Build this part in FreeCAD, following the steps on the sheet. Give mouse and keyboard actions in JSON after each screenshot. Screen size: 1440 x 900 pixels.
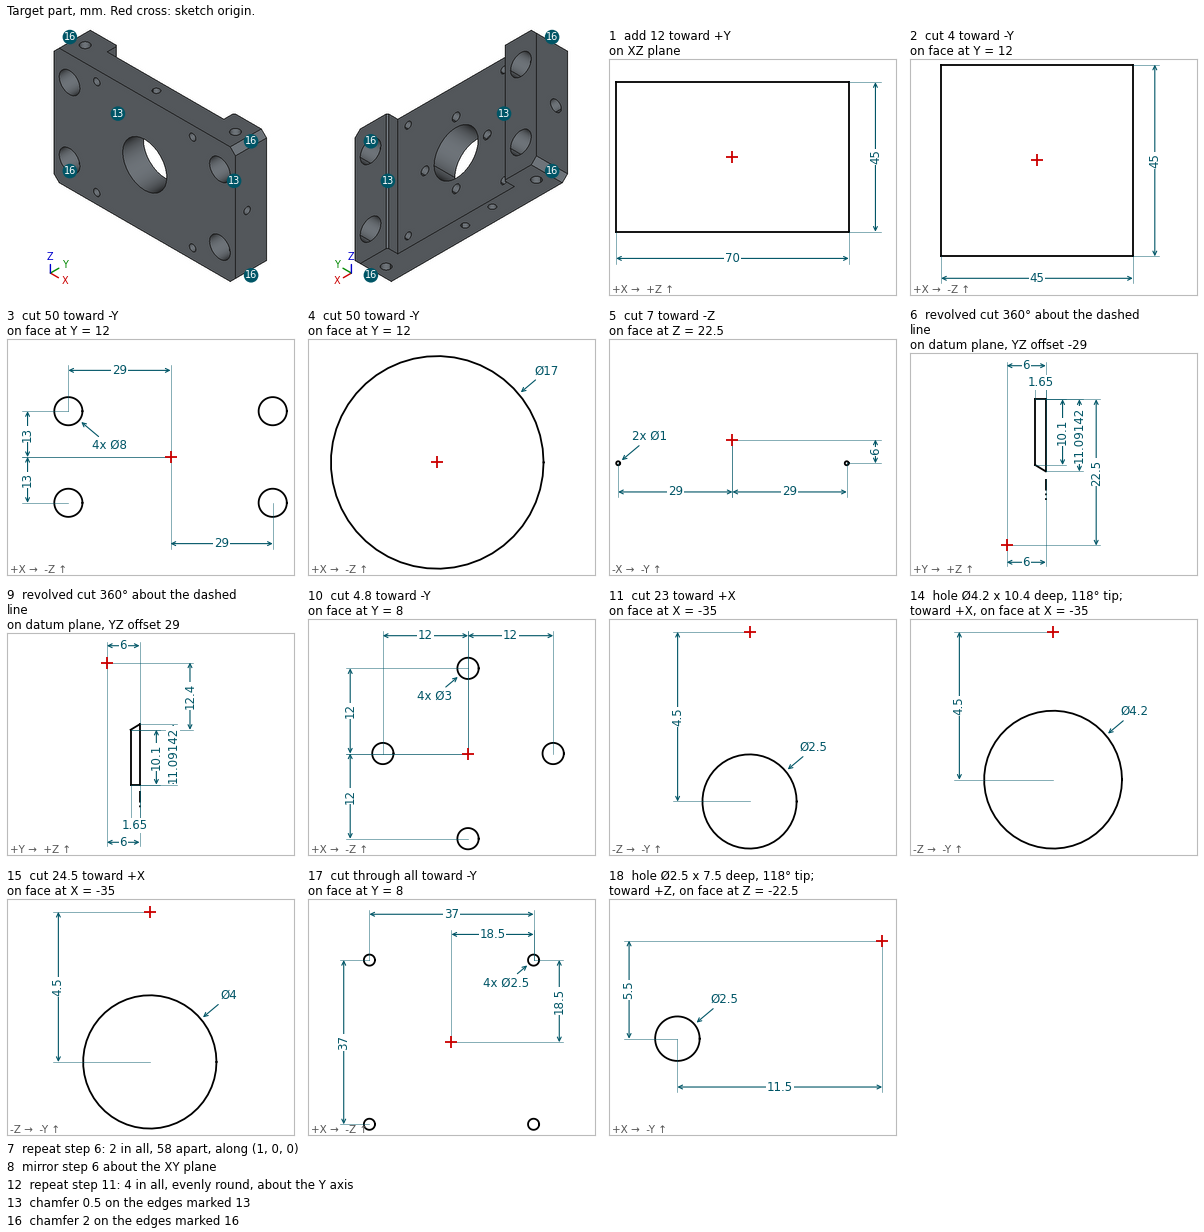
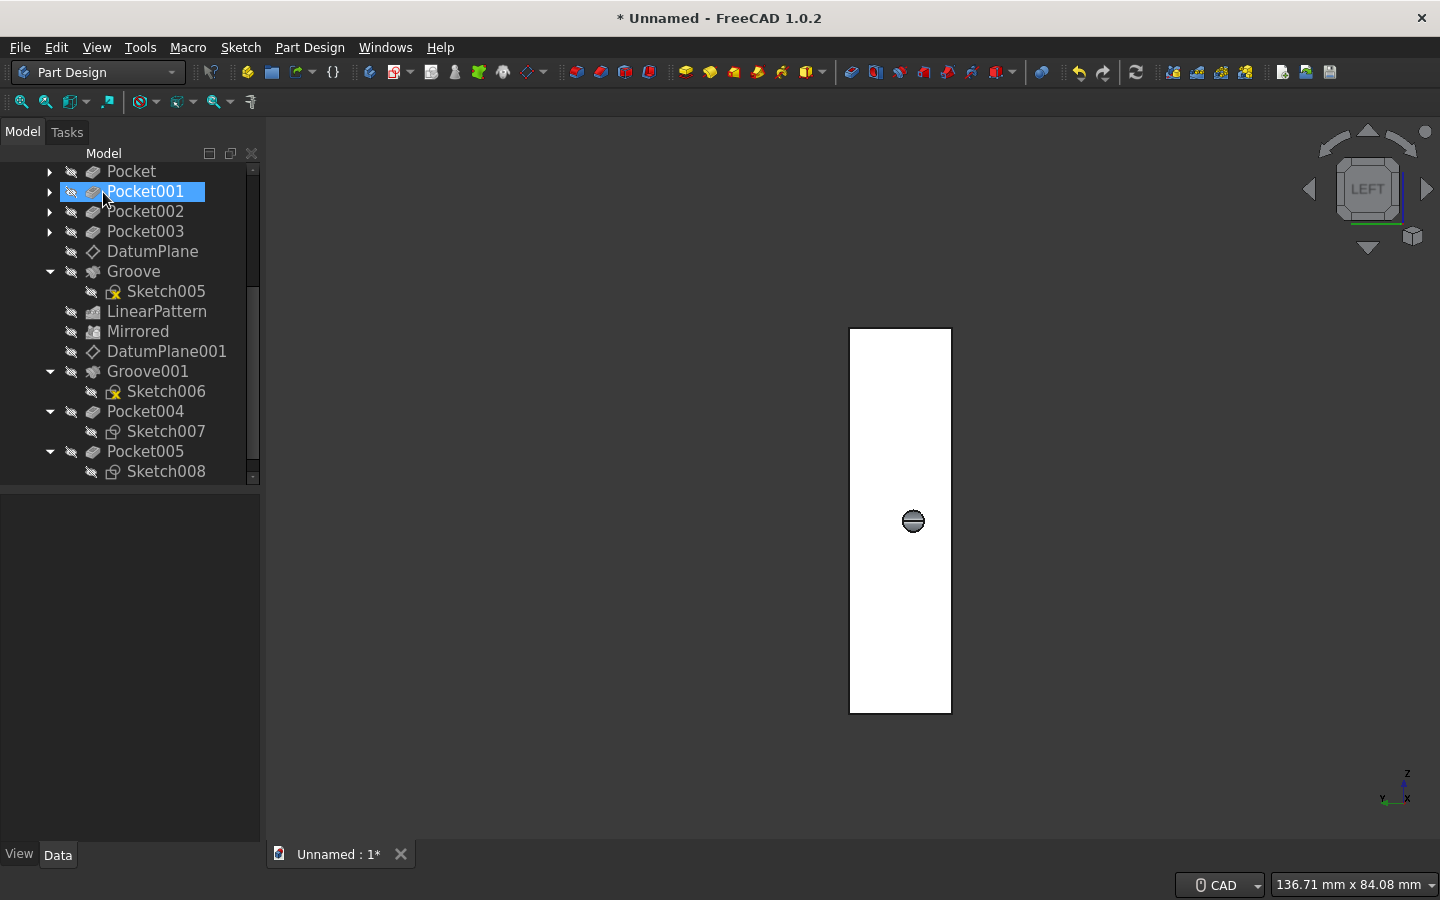
{"action": "key", "text": "0"}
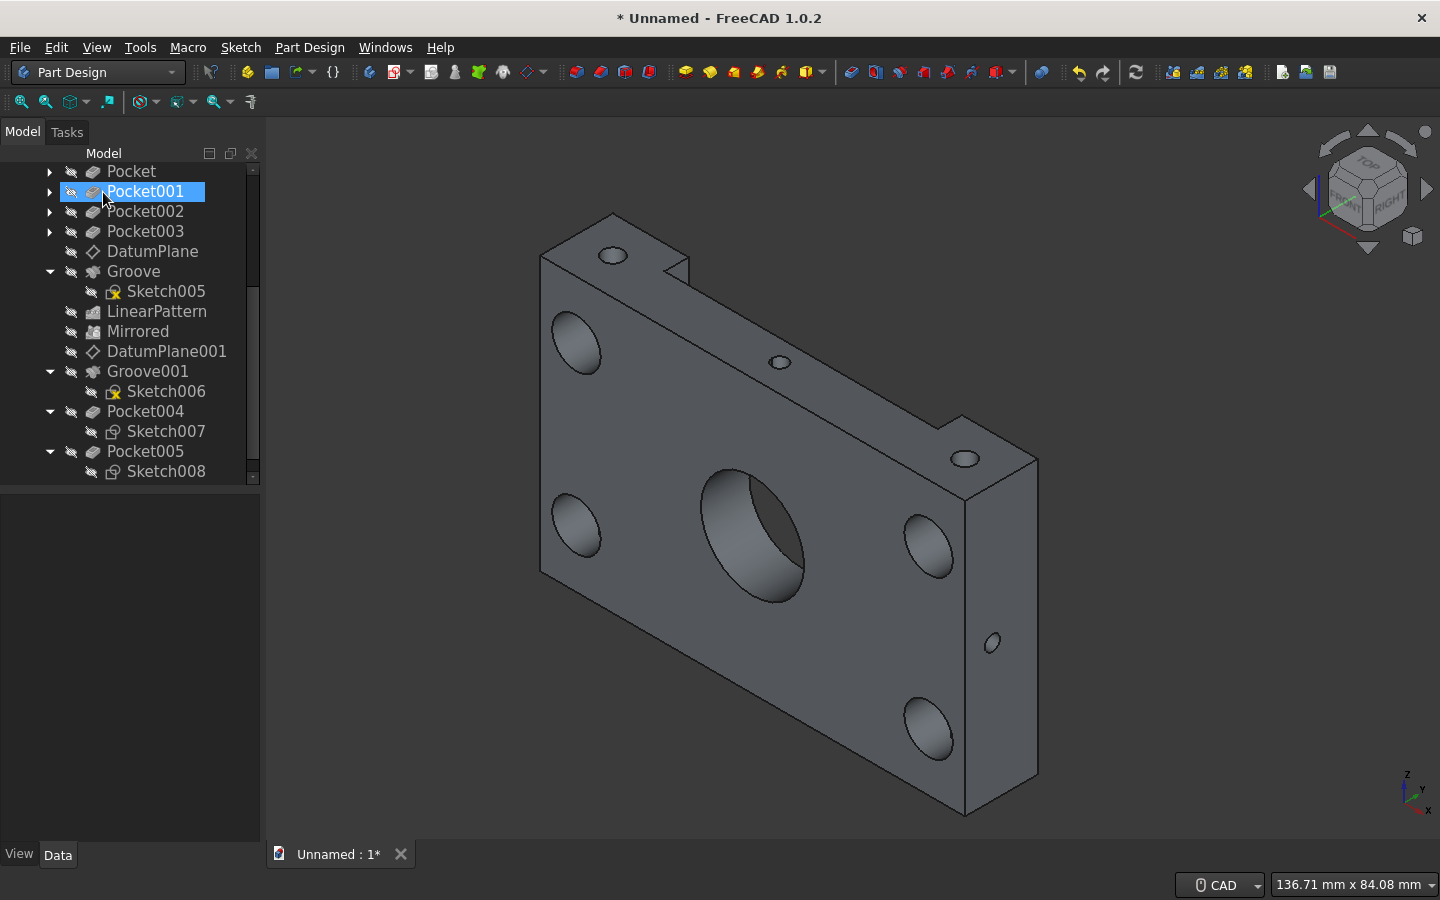
{"action": "key", "text": "2"}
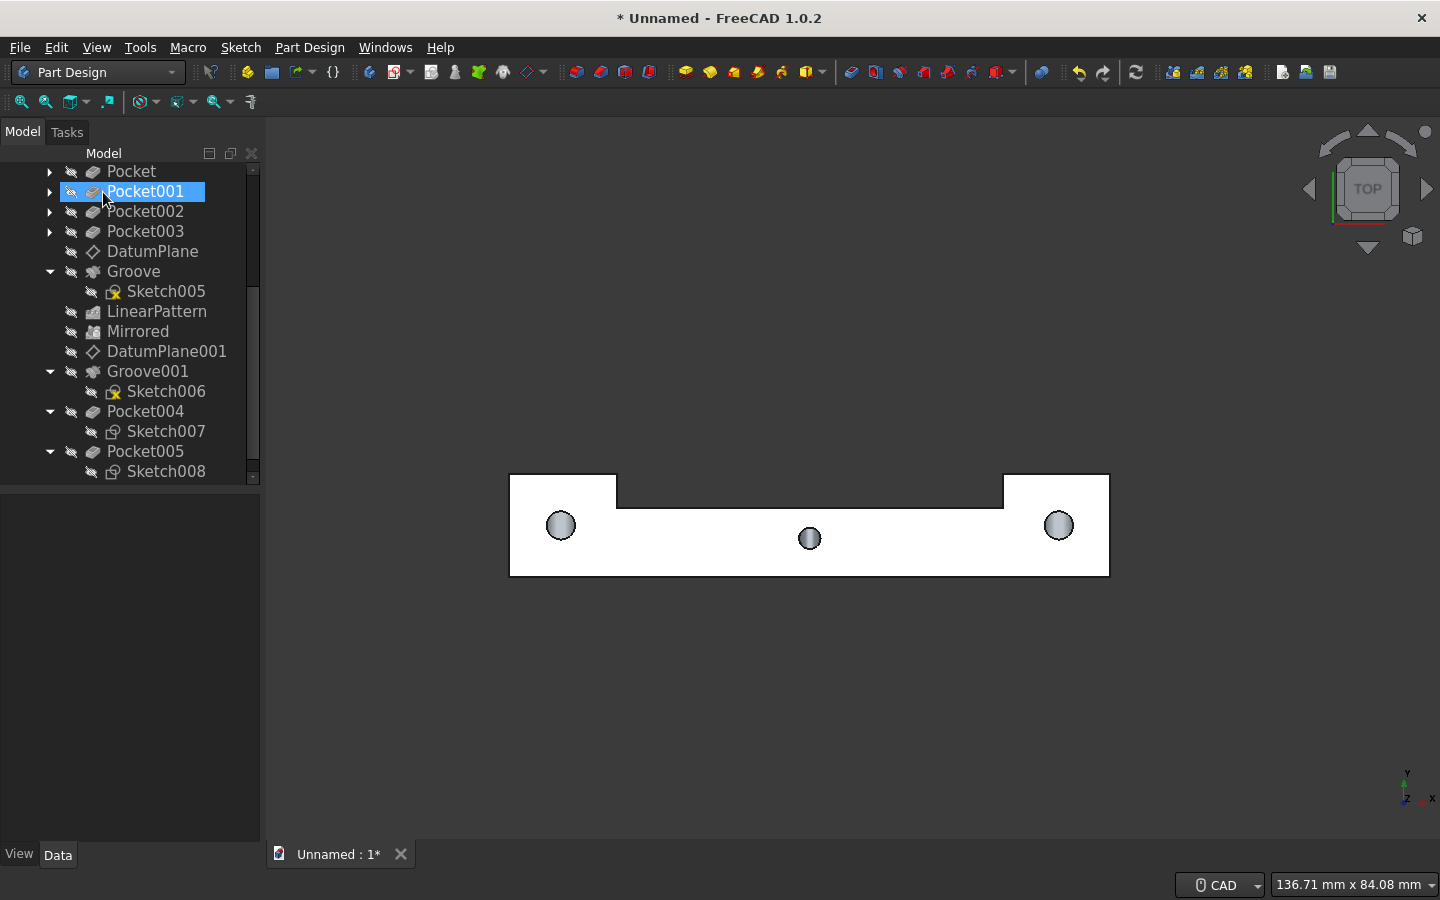
{"action": "key", "text": "1"}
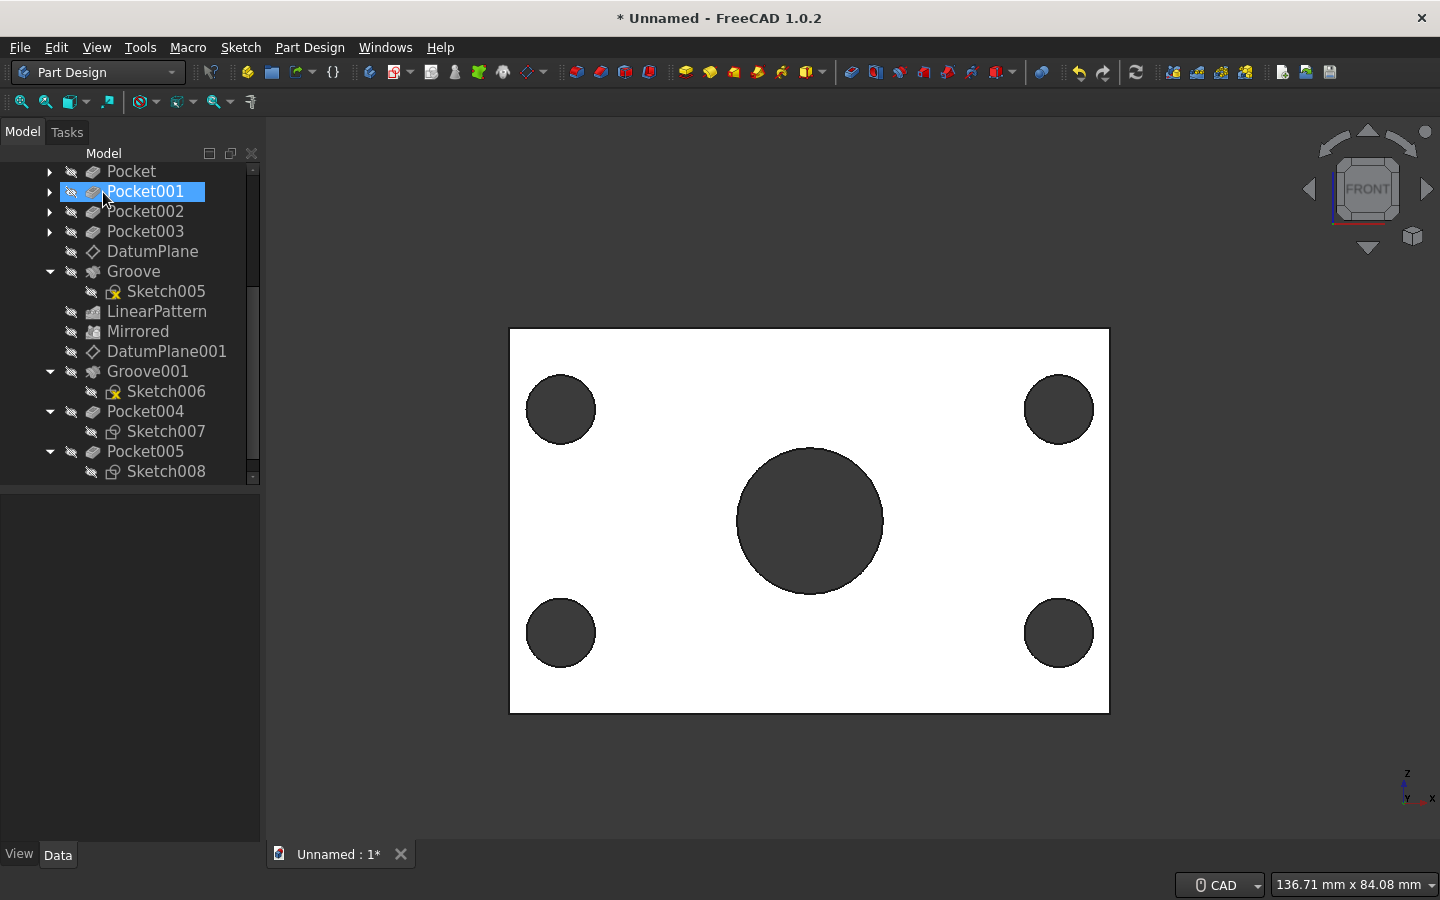
{"action": "key", "text": "3"}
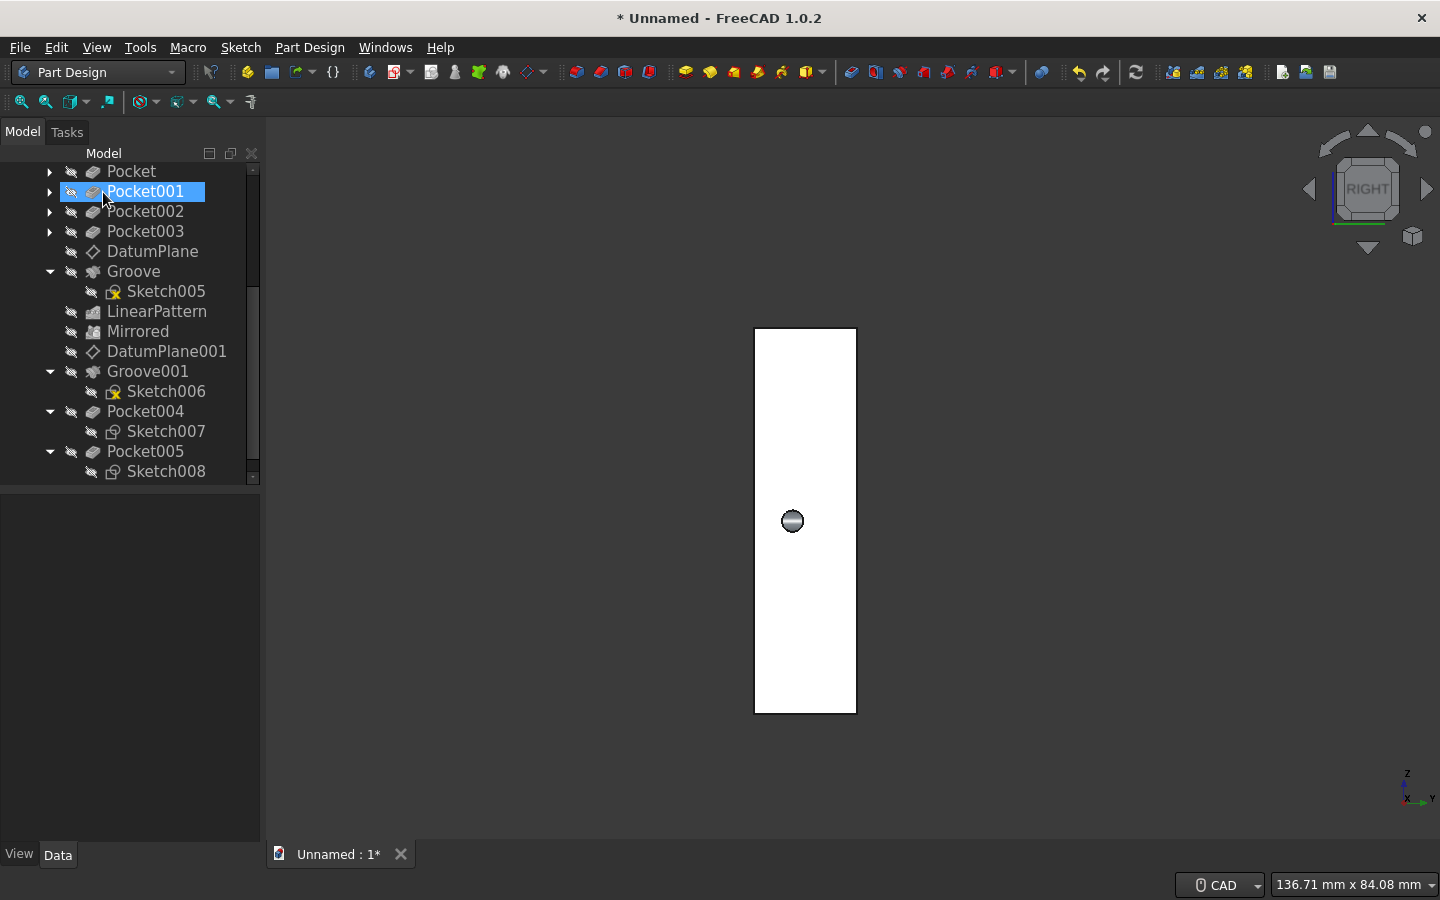
{"action": "key", "text": "5"}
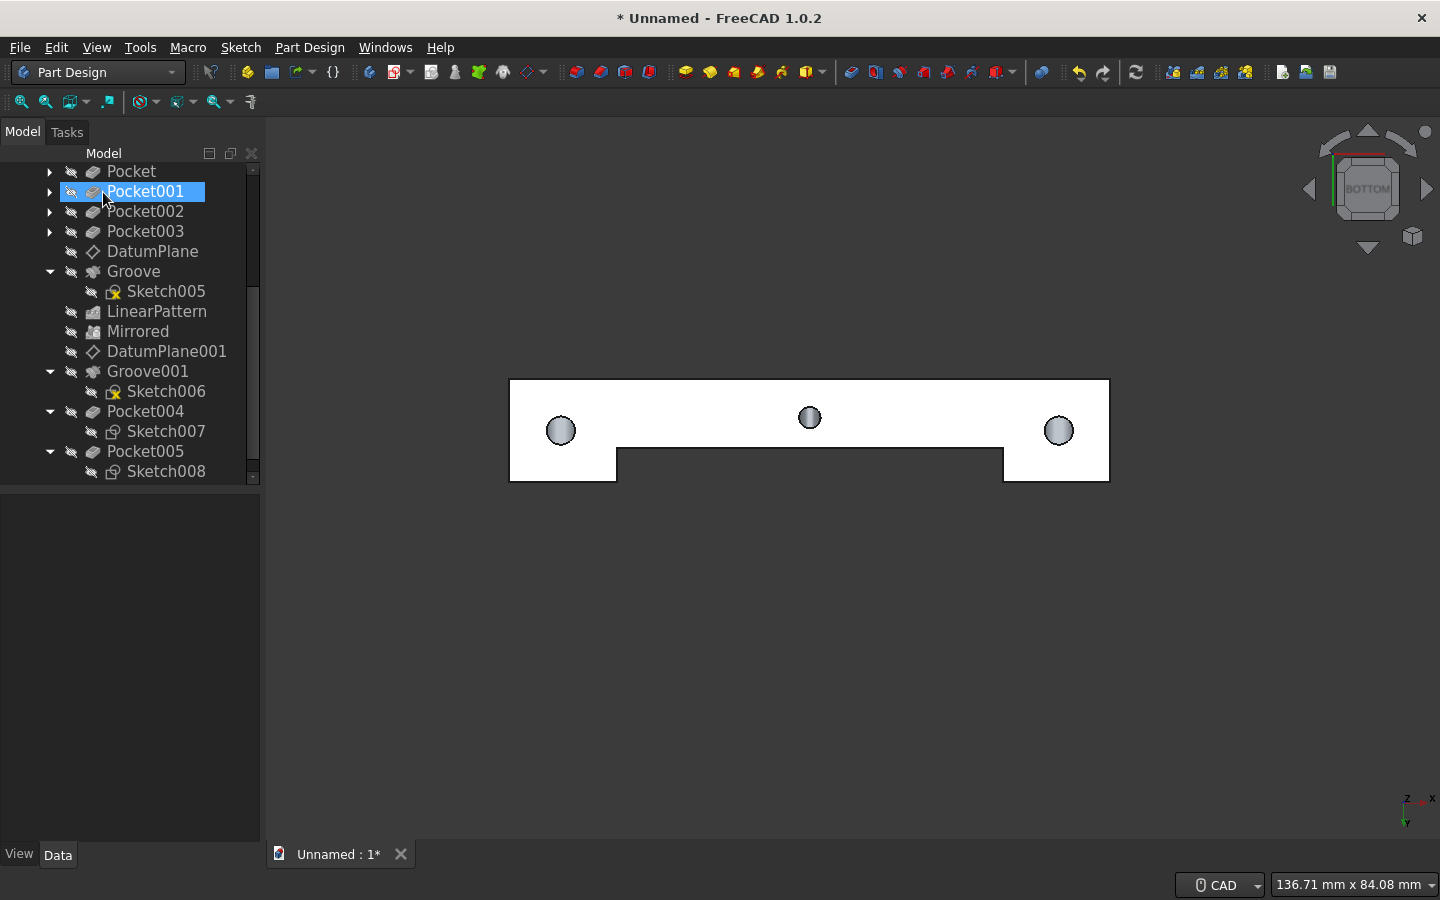
{"action": "key", "text": "4"}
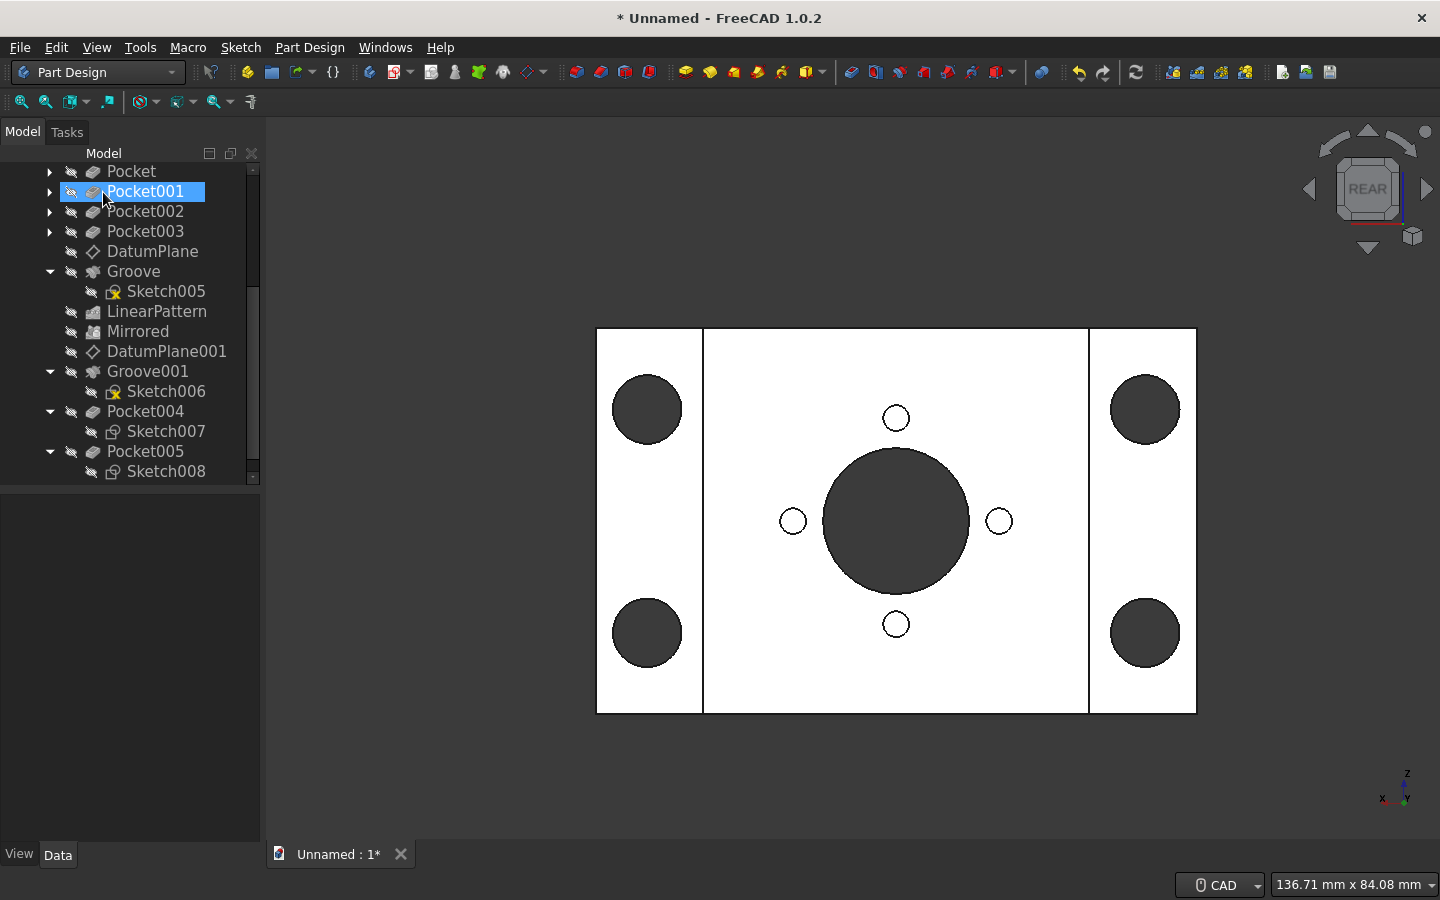
{"action": "left_click", "coordinate": [703, 520]}